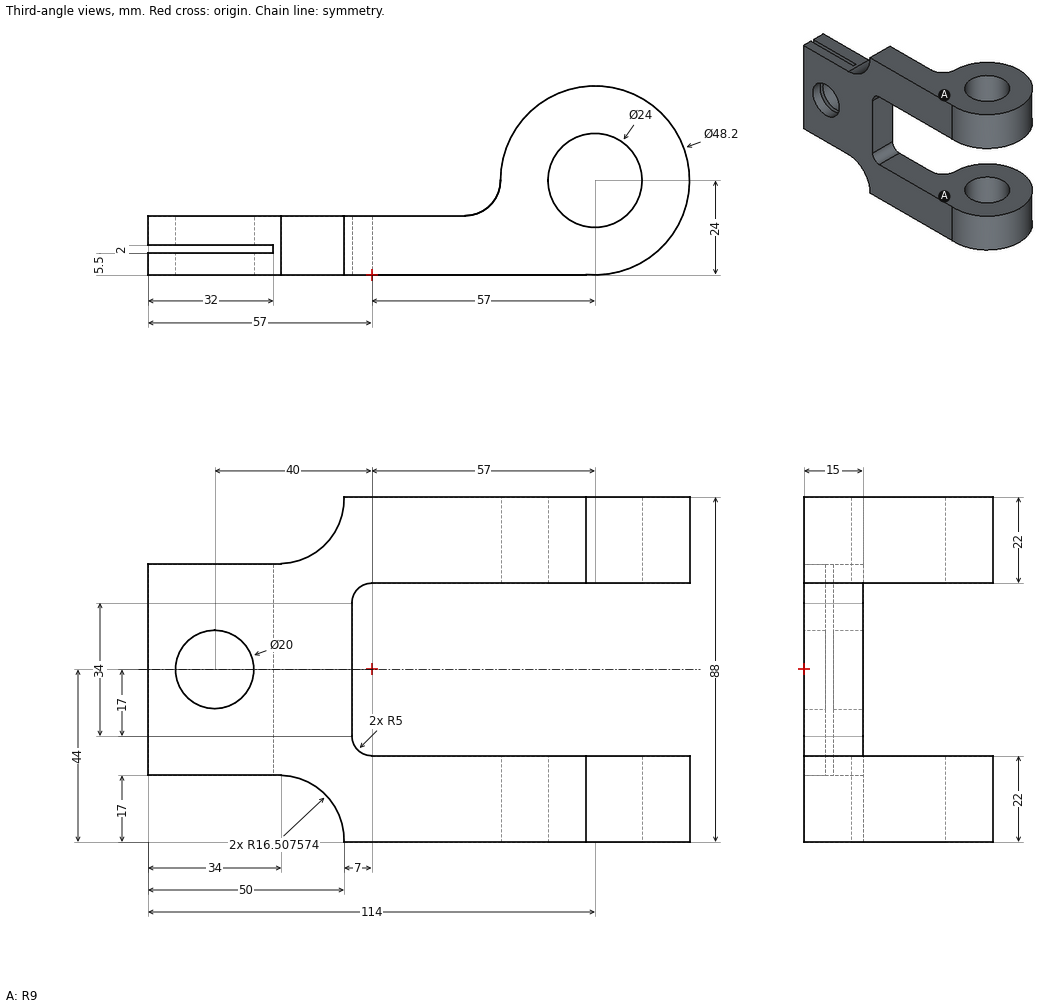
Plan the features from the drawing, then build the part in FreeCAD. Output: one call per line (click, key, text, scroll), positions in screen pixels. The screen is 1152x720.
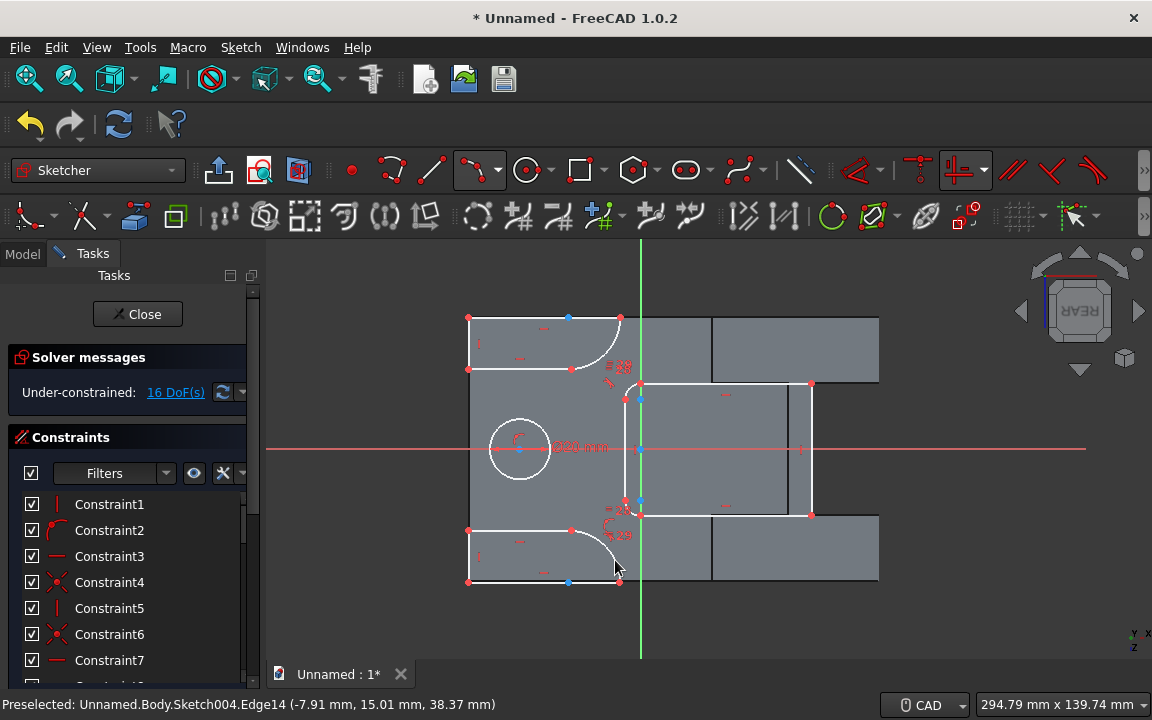
click(569, 318)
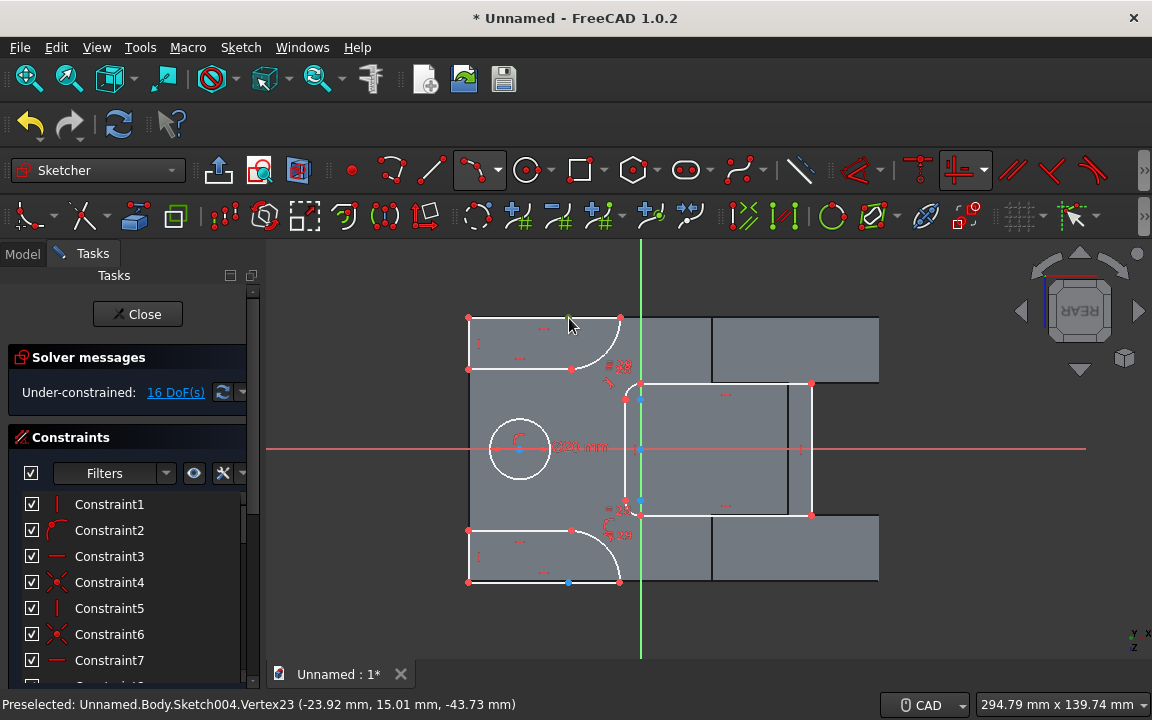
click(569, 582)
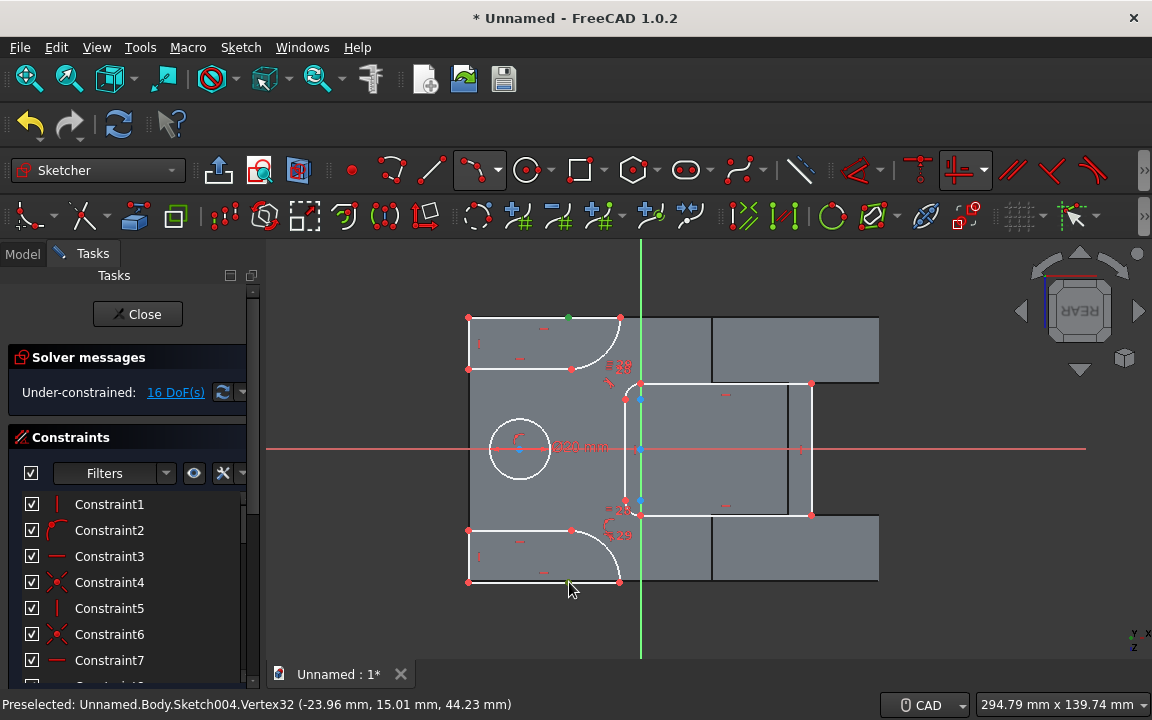
click(344, 449)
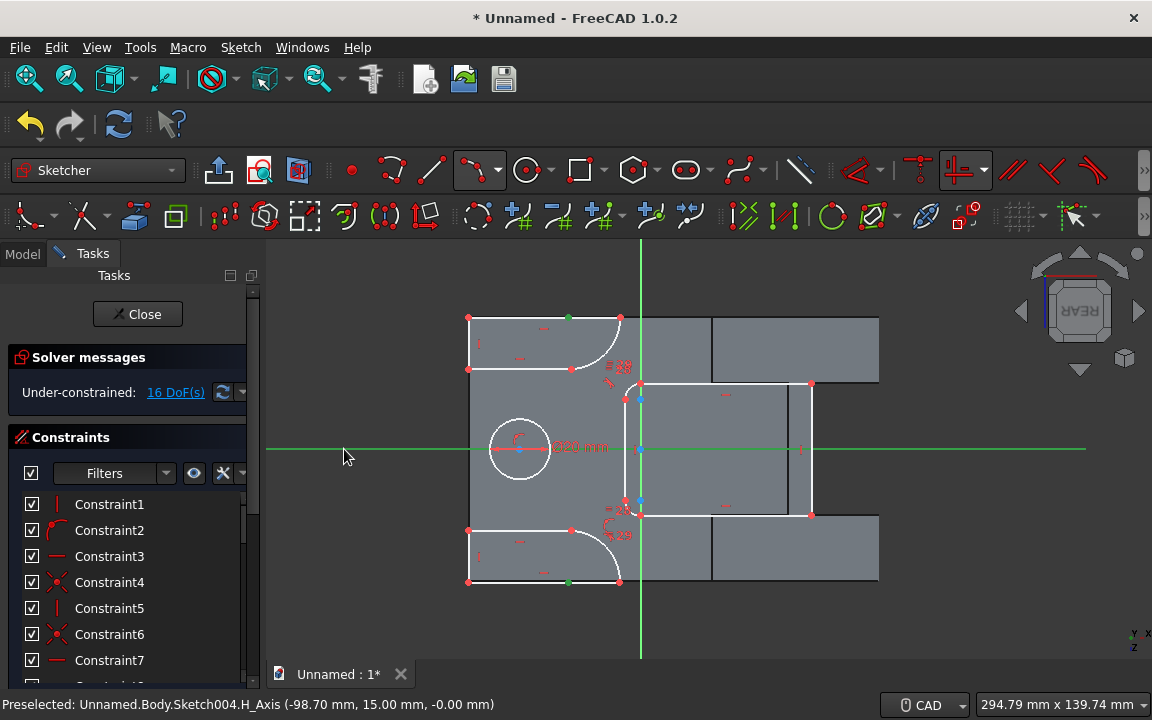
key(s)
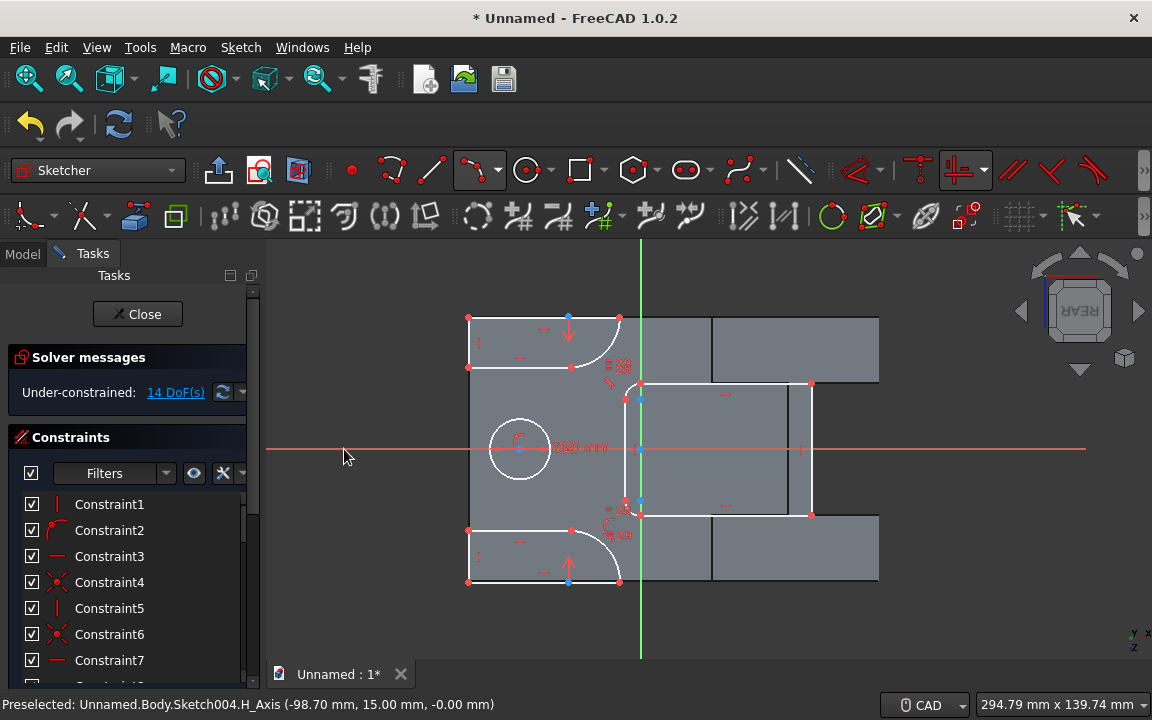
click(469, 318)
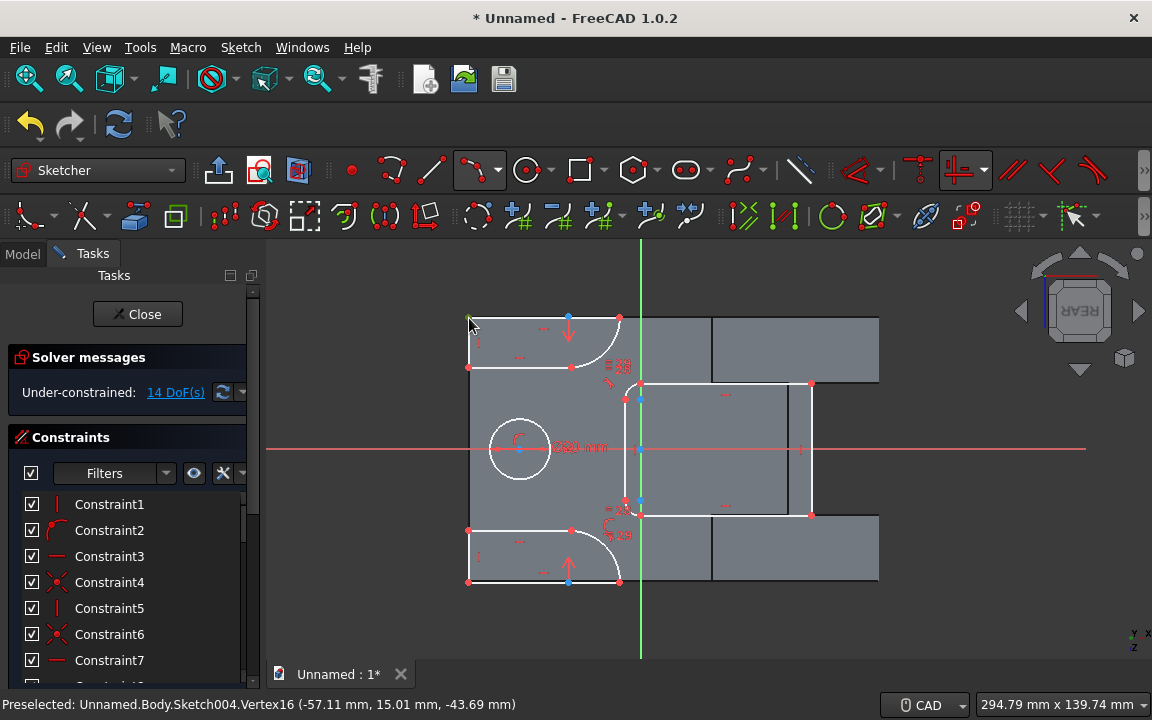
click(469, 583)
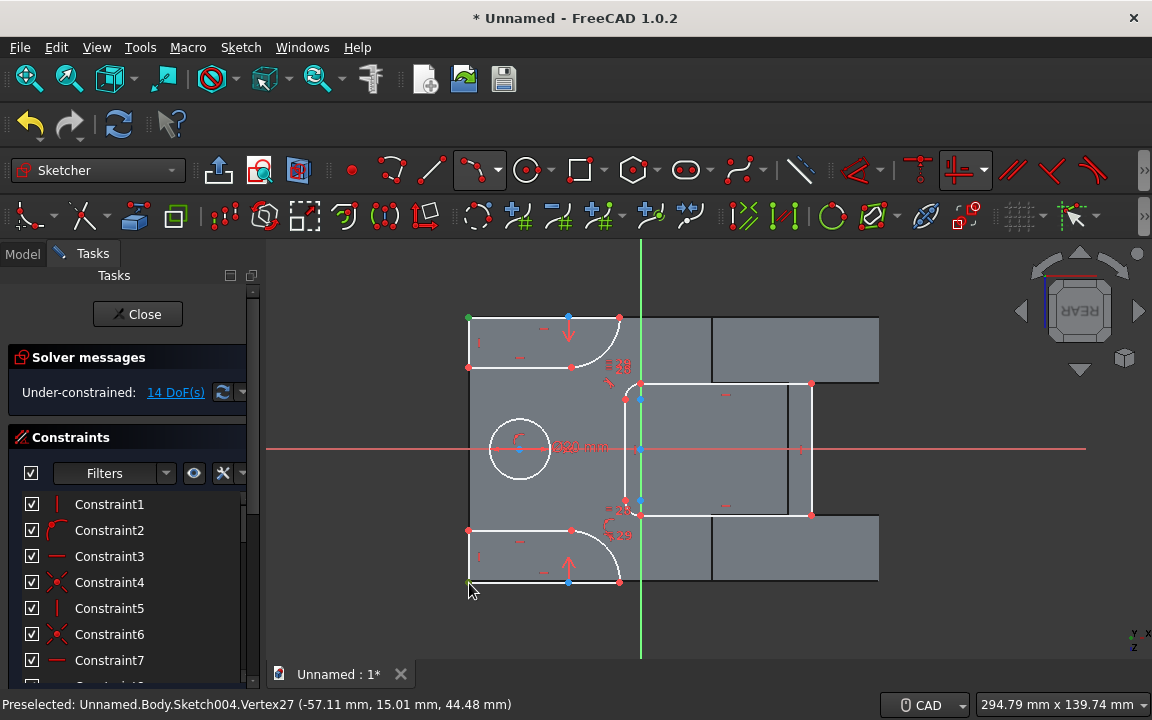
click(344, 449)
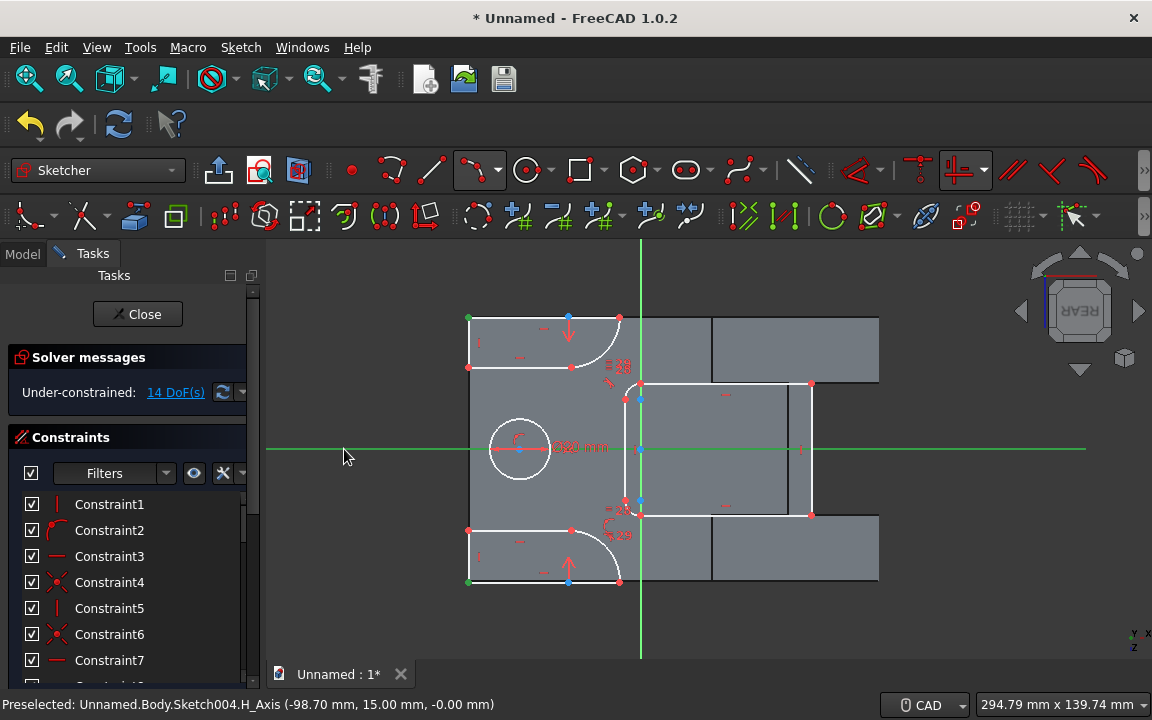
key(s)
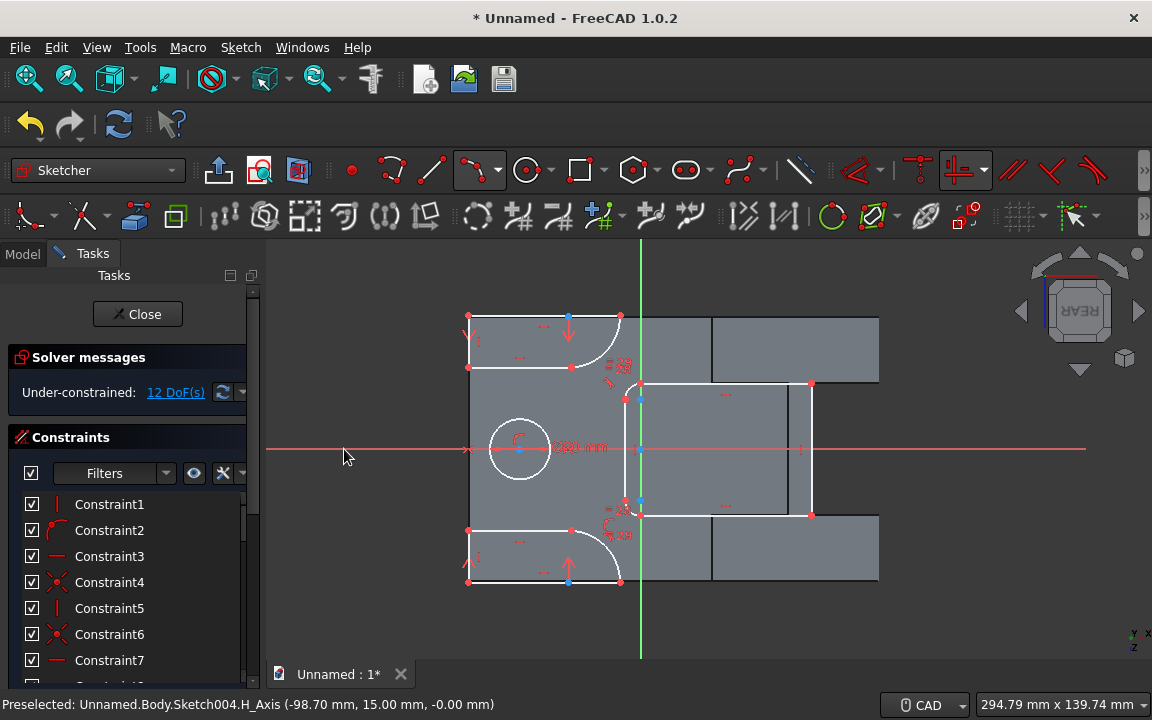
key(d)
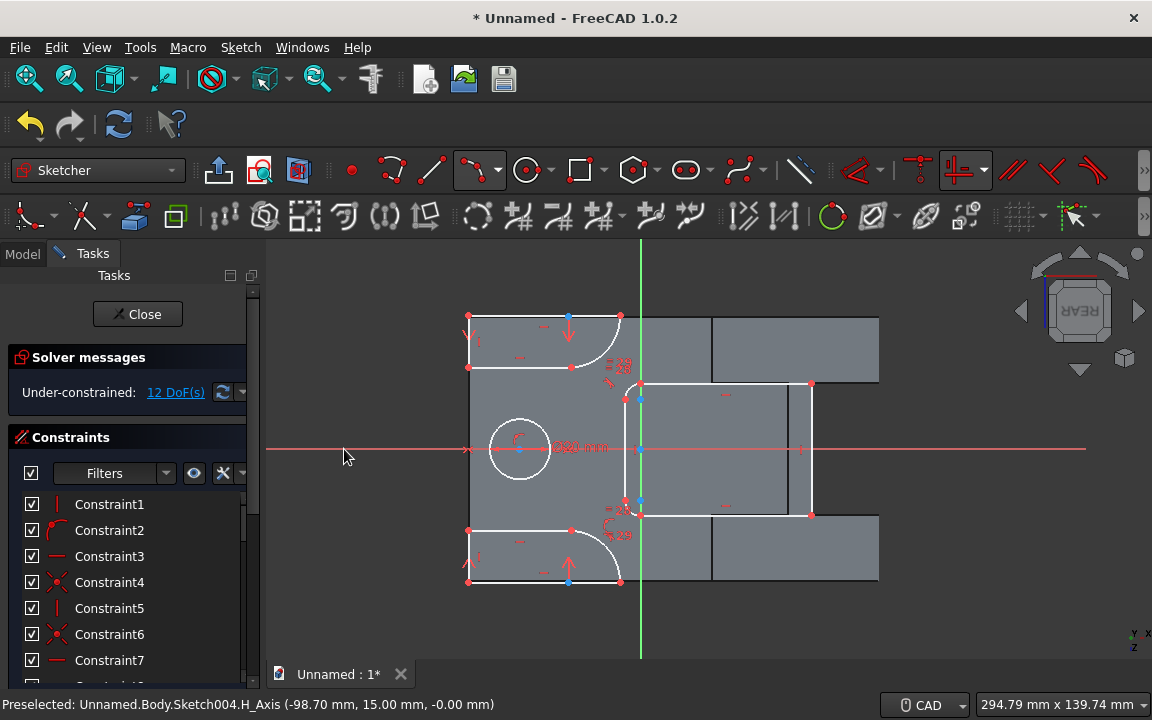
scroll(630, 511, up, 5)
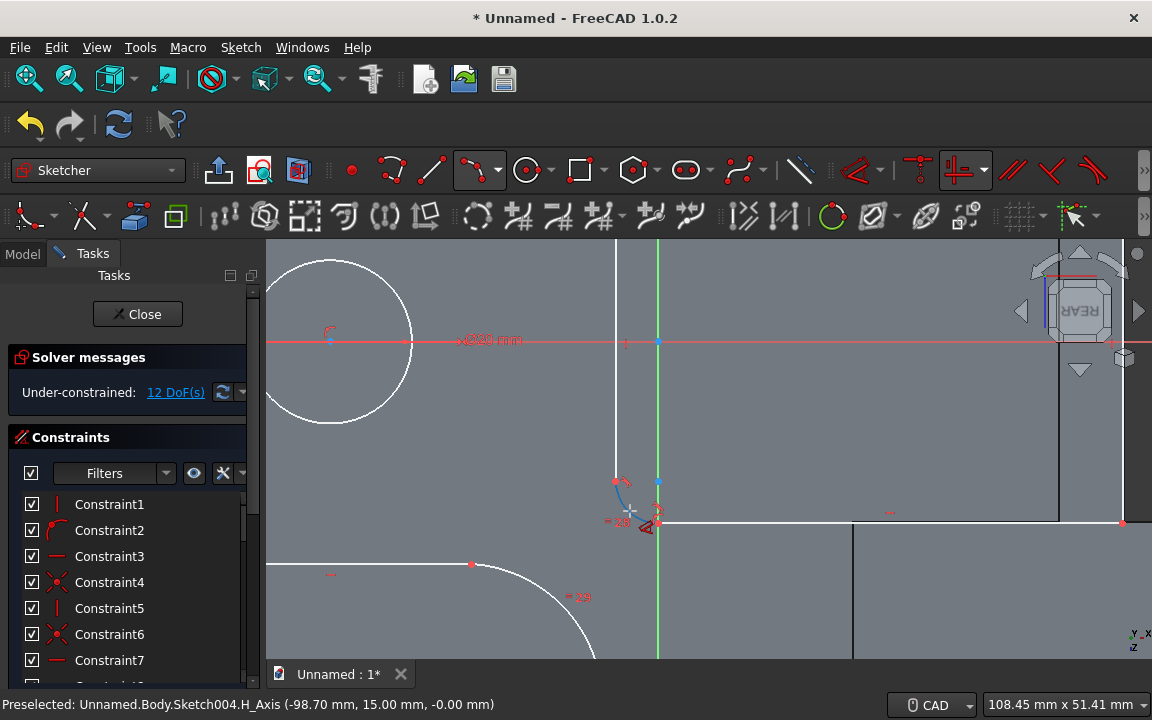
click(628, 511)
click(605, 533)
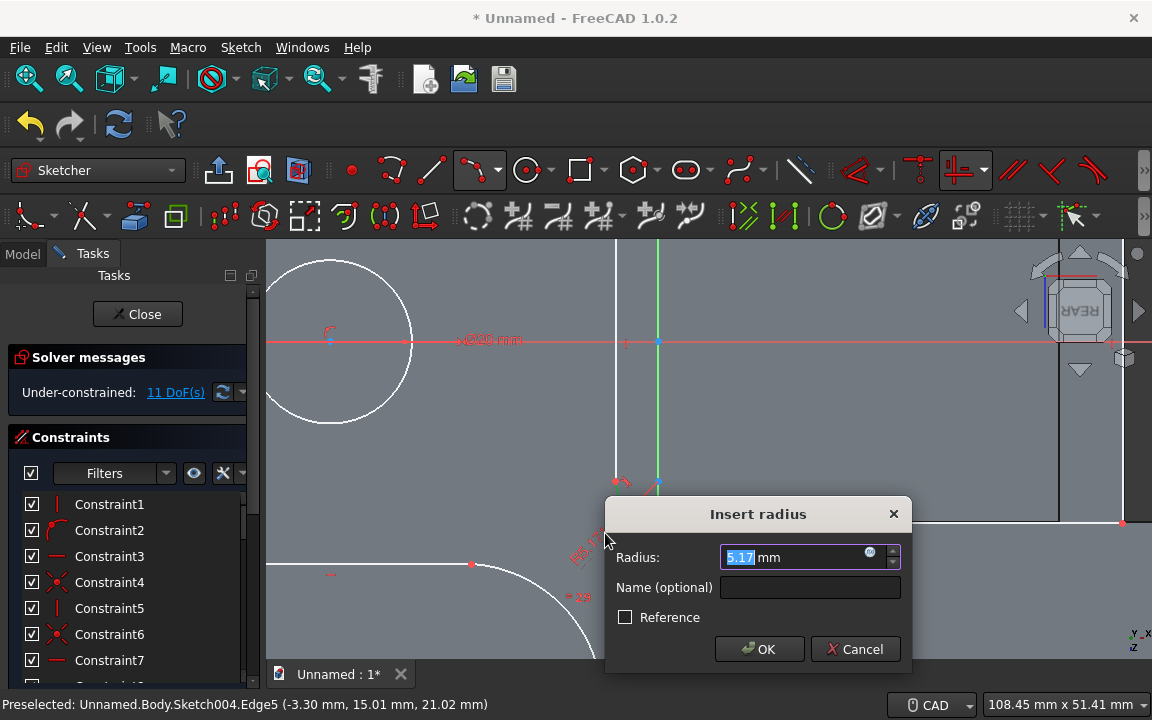
text(5)
key(Return)